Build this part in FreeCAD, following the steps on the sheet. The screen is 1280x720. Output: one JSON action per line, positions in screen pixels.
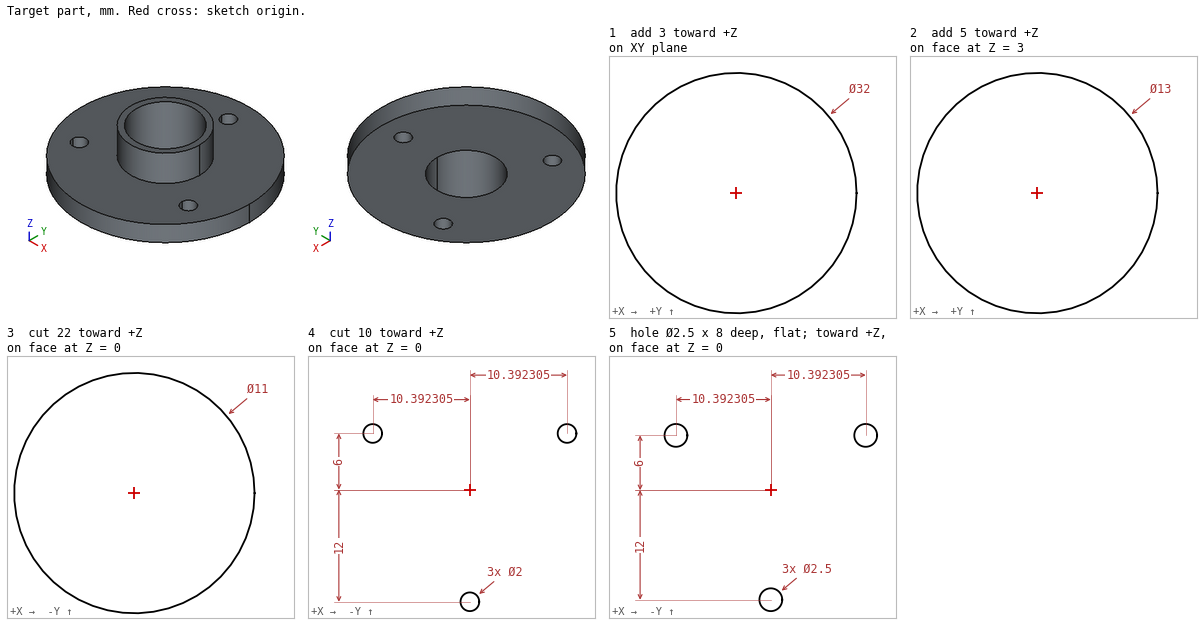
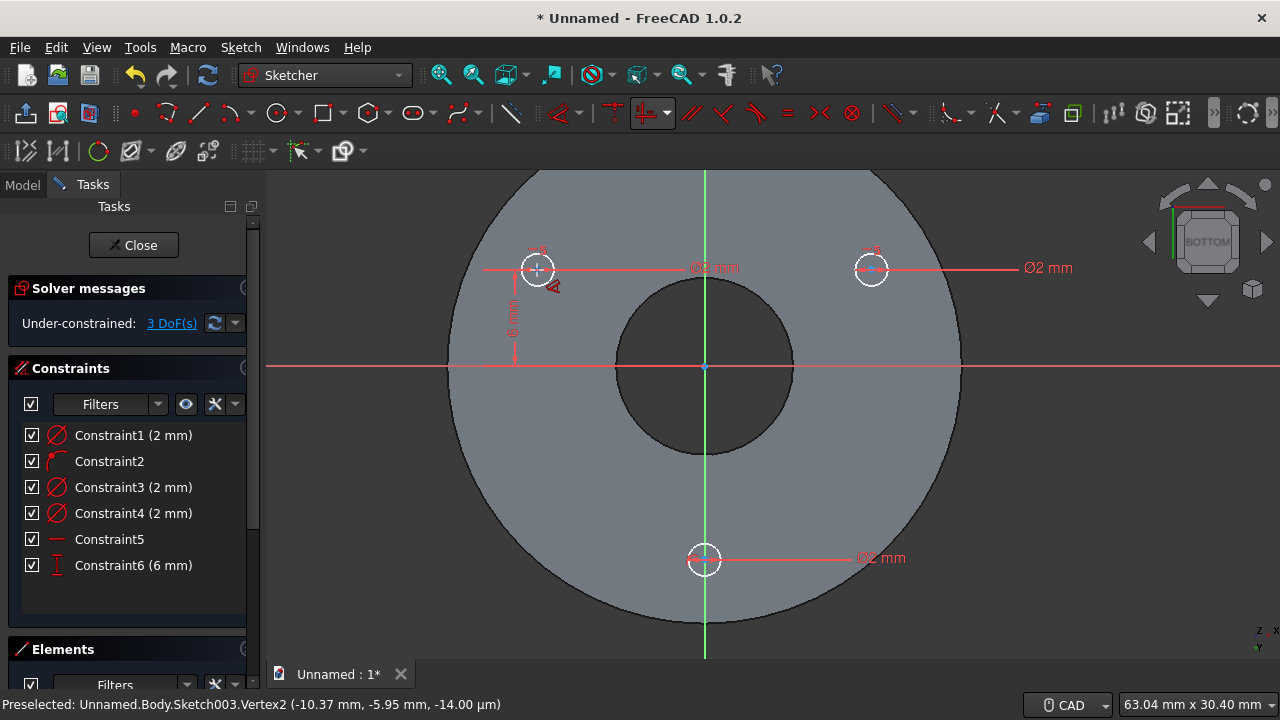
{"action": "left_click", "coordinate": [705, 560]}
{"action": "left_click", "coordinate": [739, 463]}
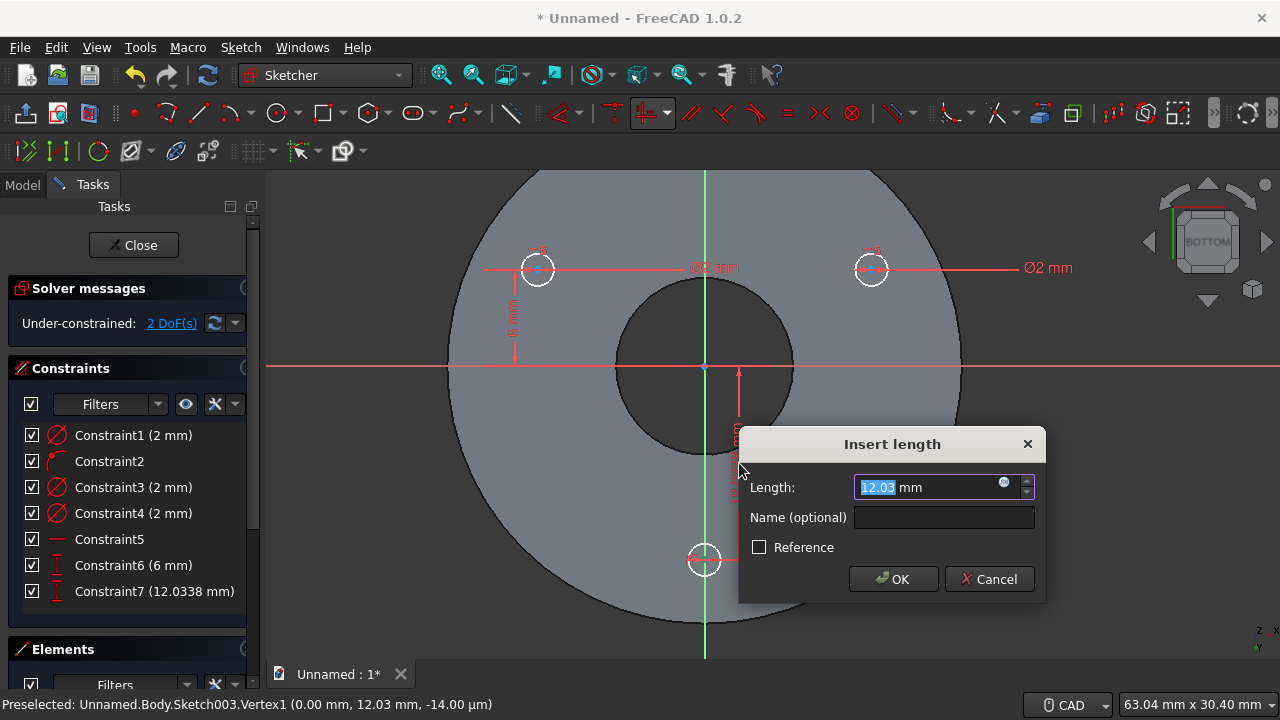
{"action": "type", "text": "12"}
{"action": "key", "text": "Return"}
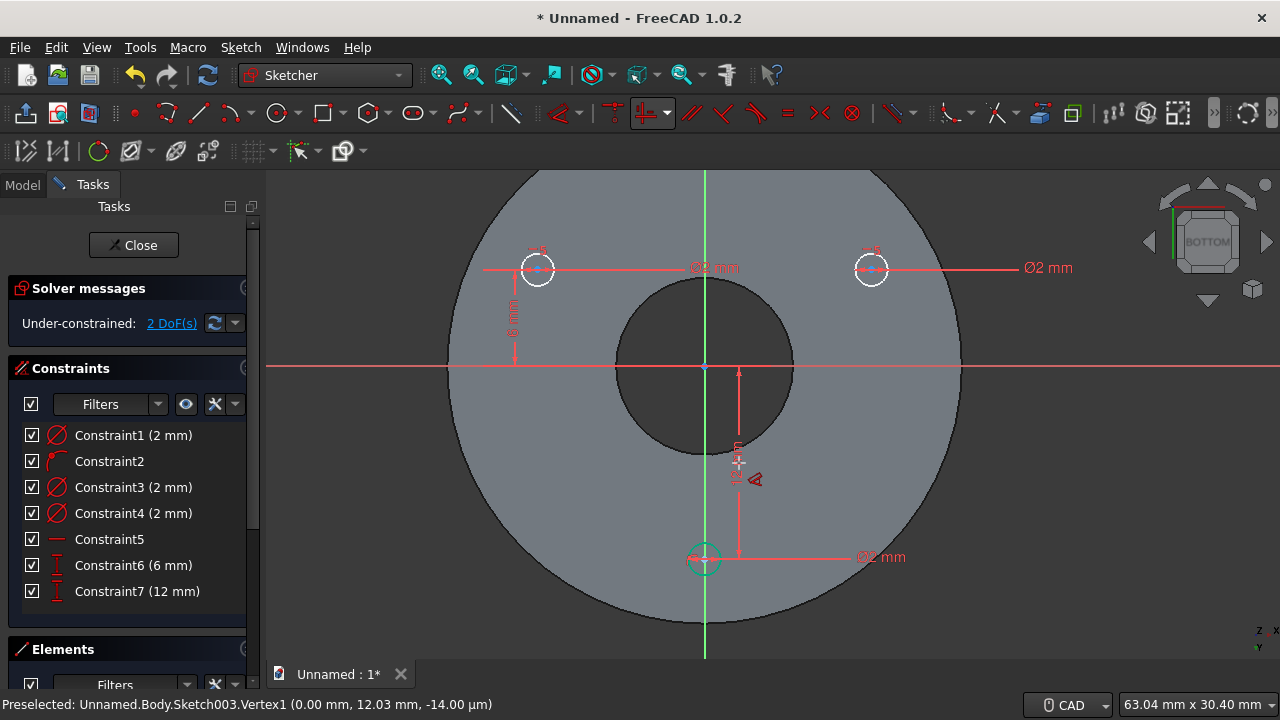
{"action": "left_click", "coordinate": [538, 270]}
{"action": "left_click", "coordinate": [621, 236]}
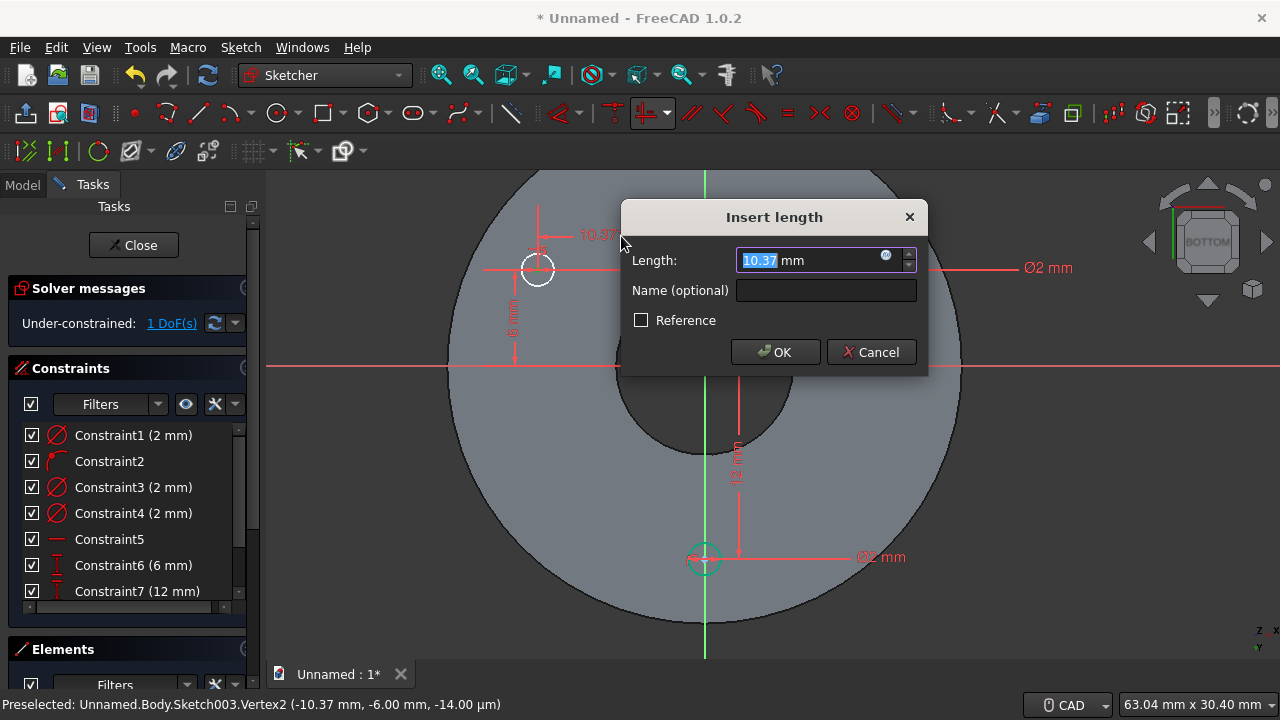
{"action": "type", "text": "10.392305"}
{"action": "key", "text": "Return"}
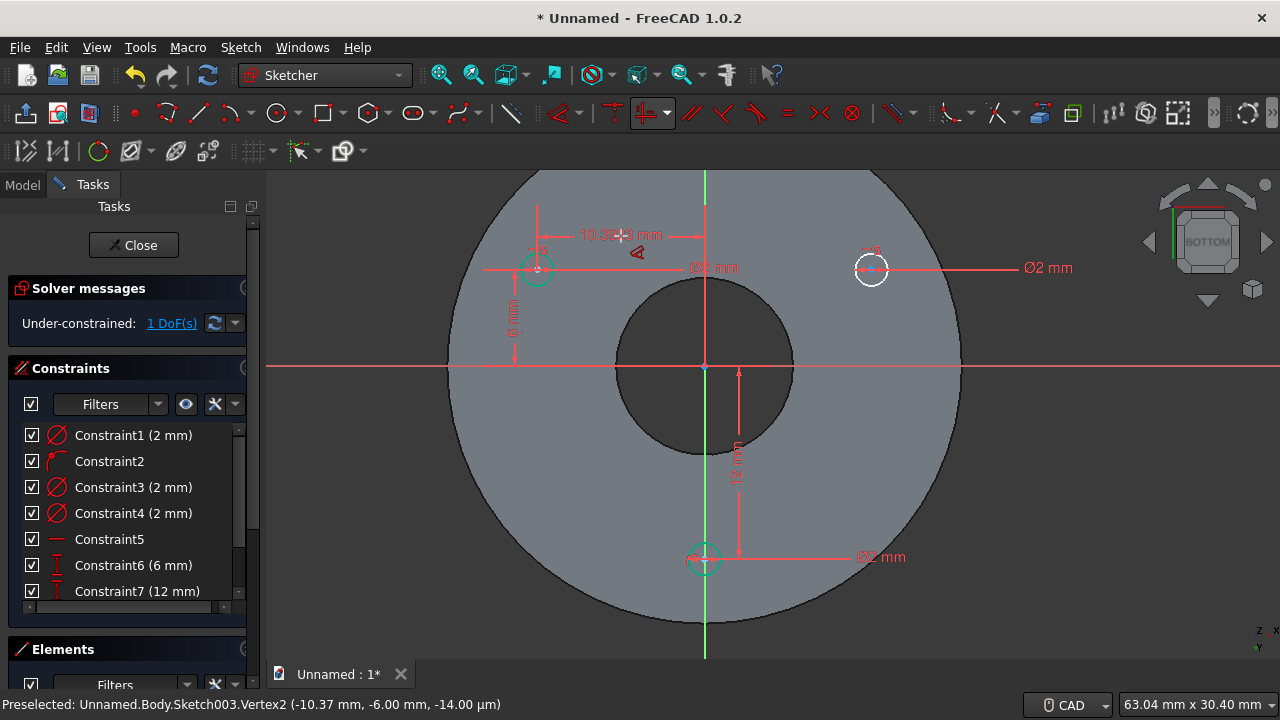
{"action": "left_click", "coordinate": [872, 270]}
{"action": "left_click", "coordinate": [788, 236]}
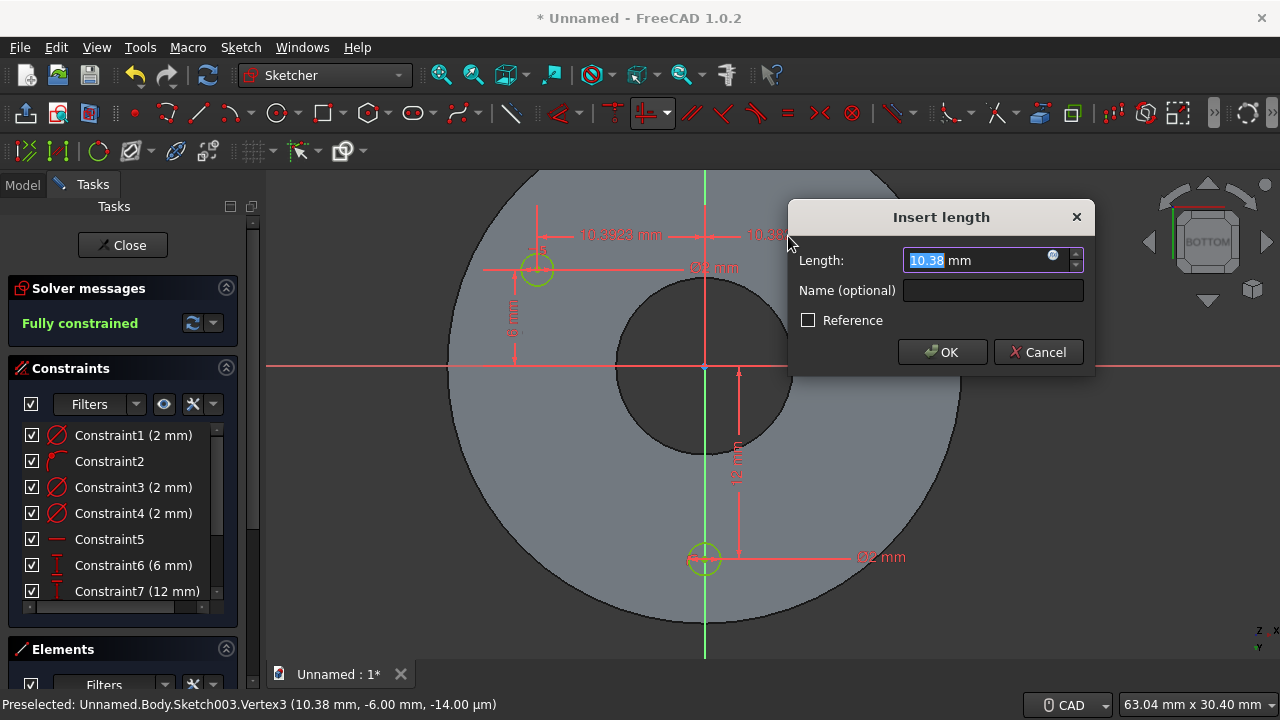
{"action": "type", "text": "10.392305"}
{"action": "key", "text": "Return"}
{"action": "key", "text": "Escape"}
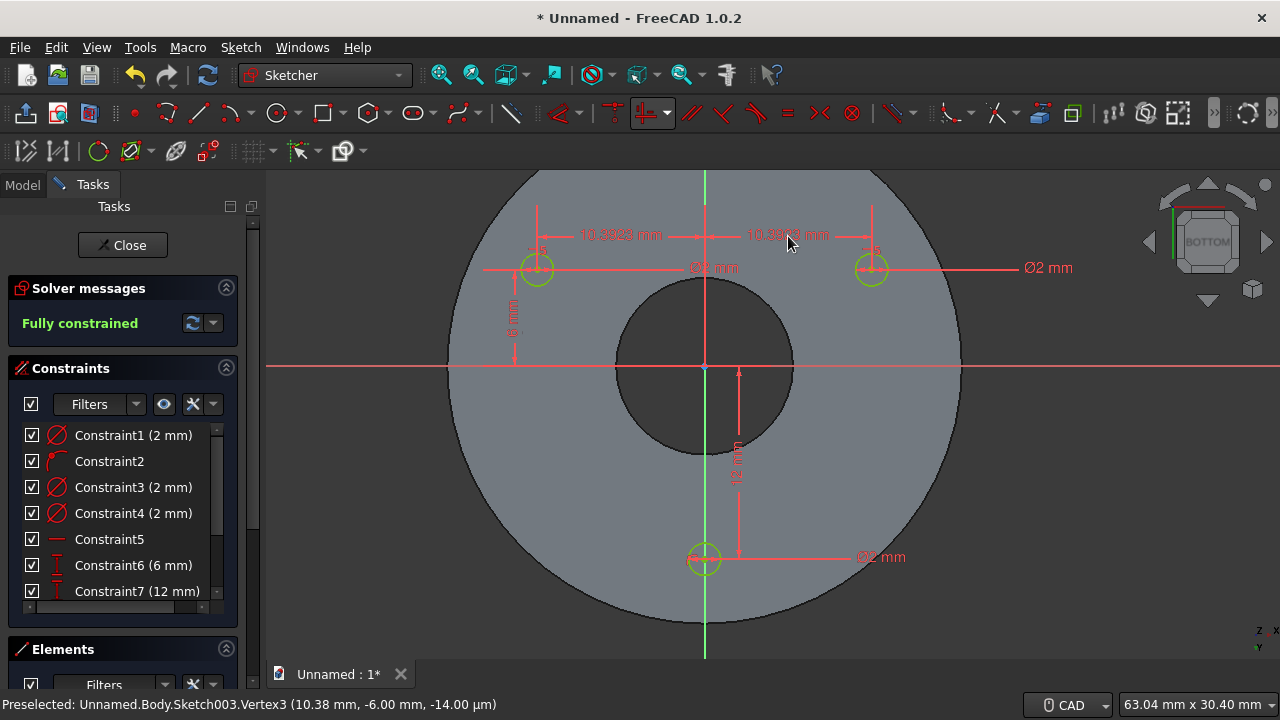
{"action": "left_click", "coordinate": [123, 245]}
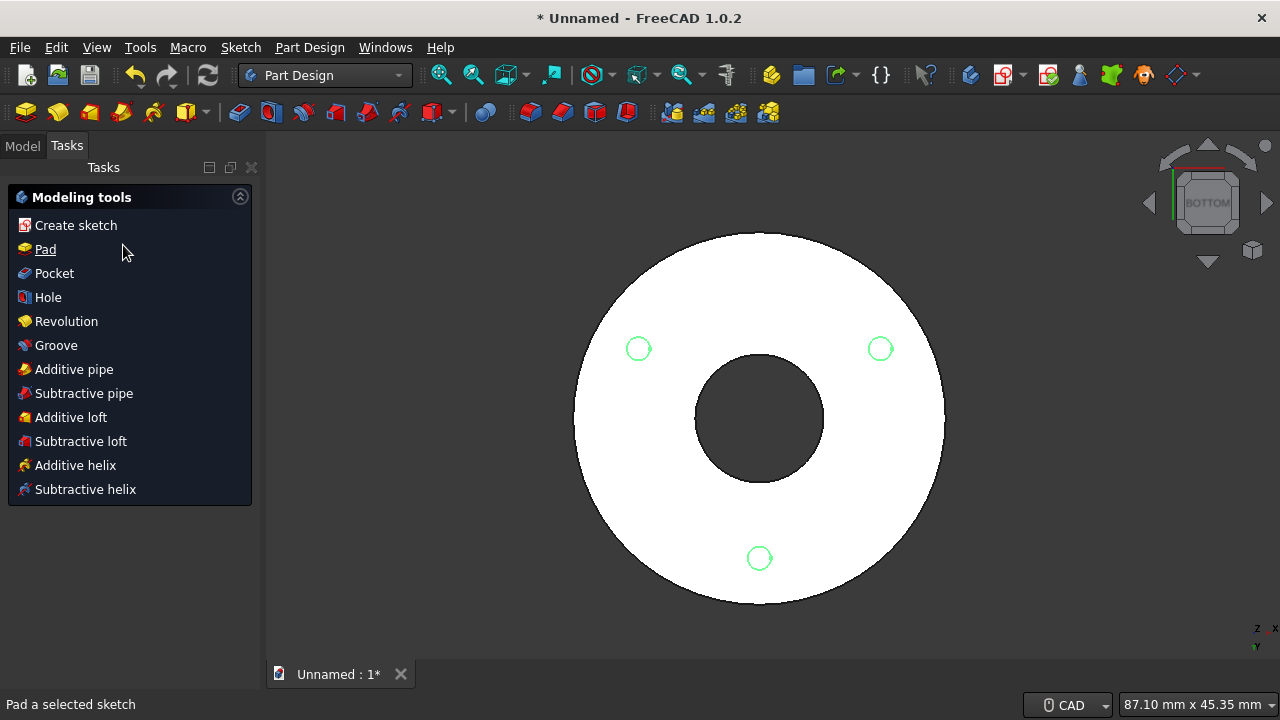
{"action": "left_click", "coordinate": [240, 112]}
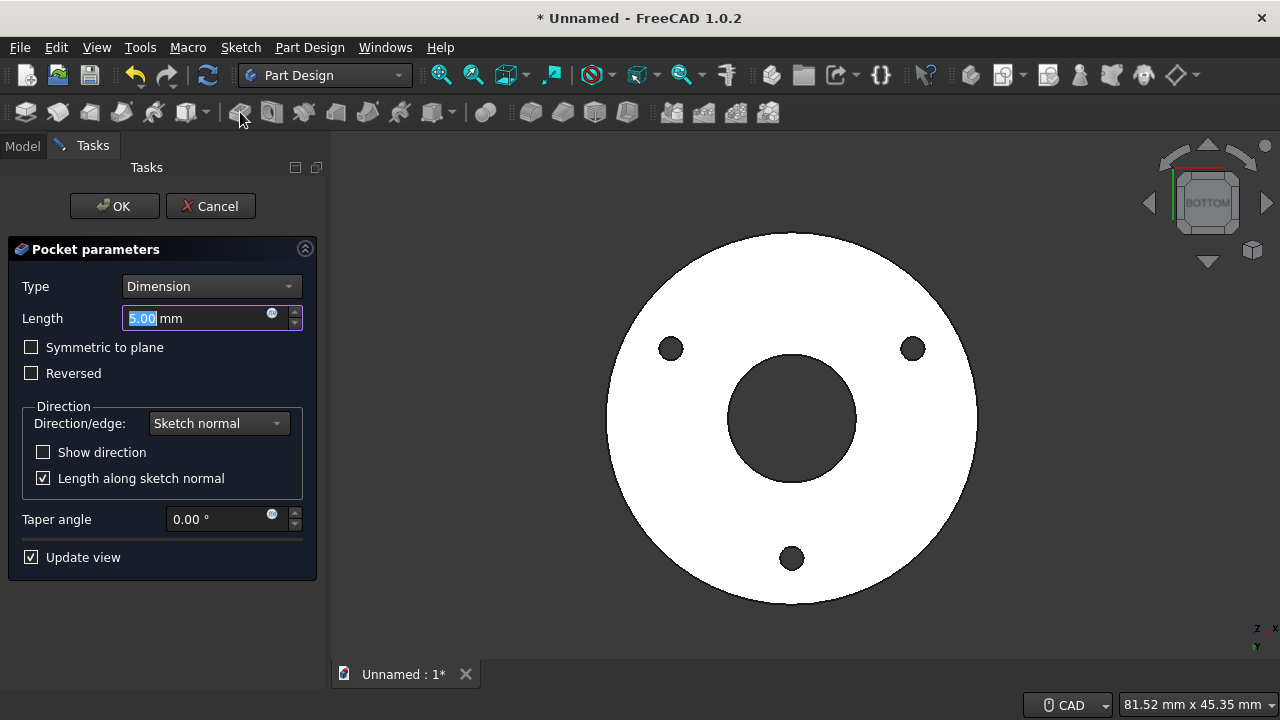
{"action": "type", "text": "10"}
{"action": "key", "text": "Tab"}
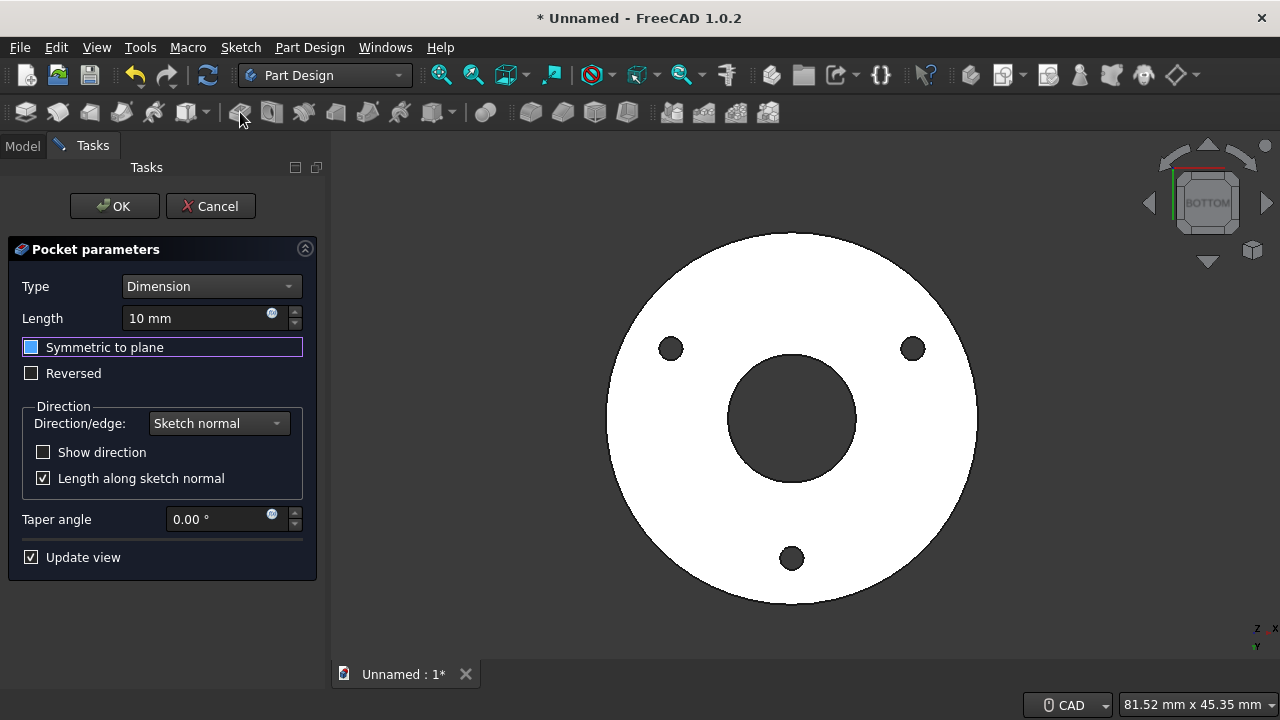
{"action": "left_click", "coordinate": [115, 206]}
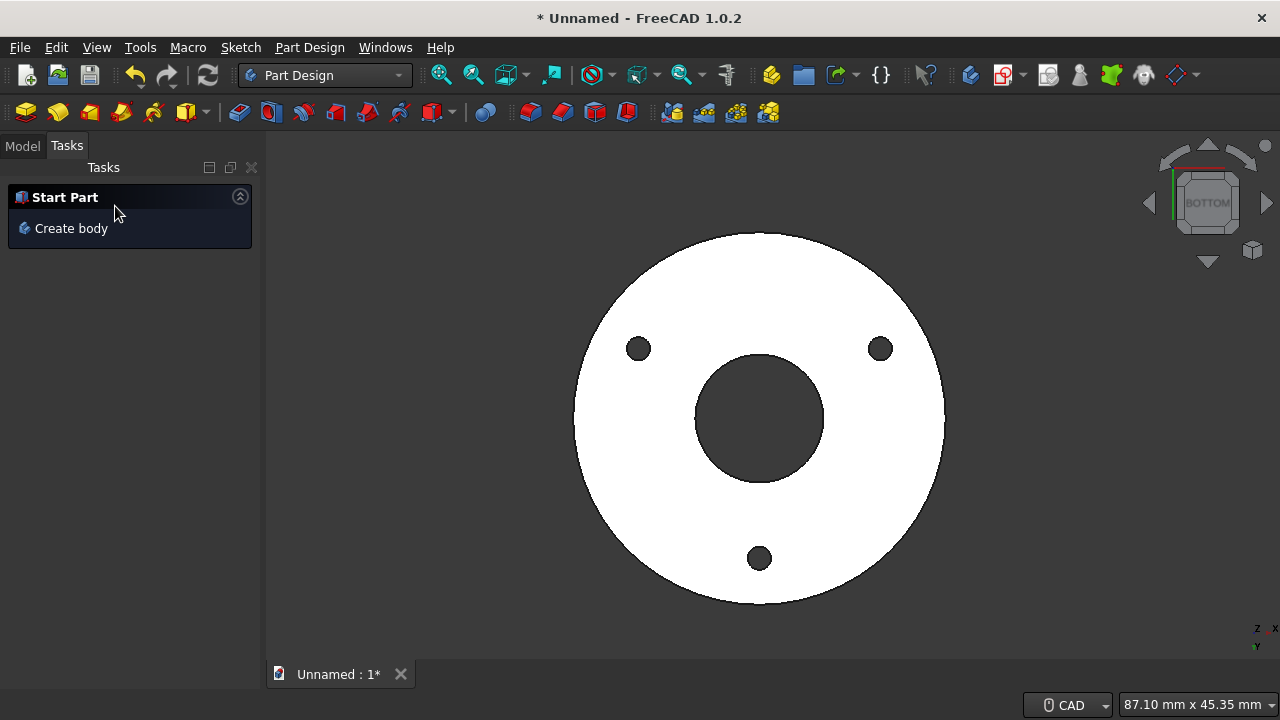
{"action": "left_click", "coordinate": [653, 471]}